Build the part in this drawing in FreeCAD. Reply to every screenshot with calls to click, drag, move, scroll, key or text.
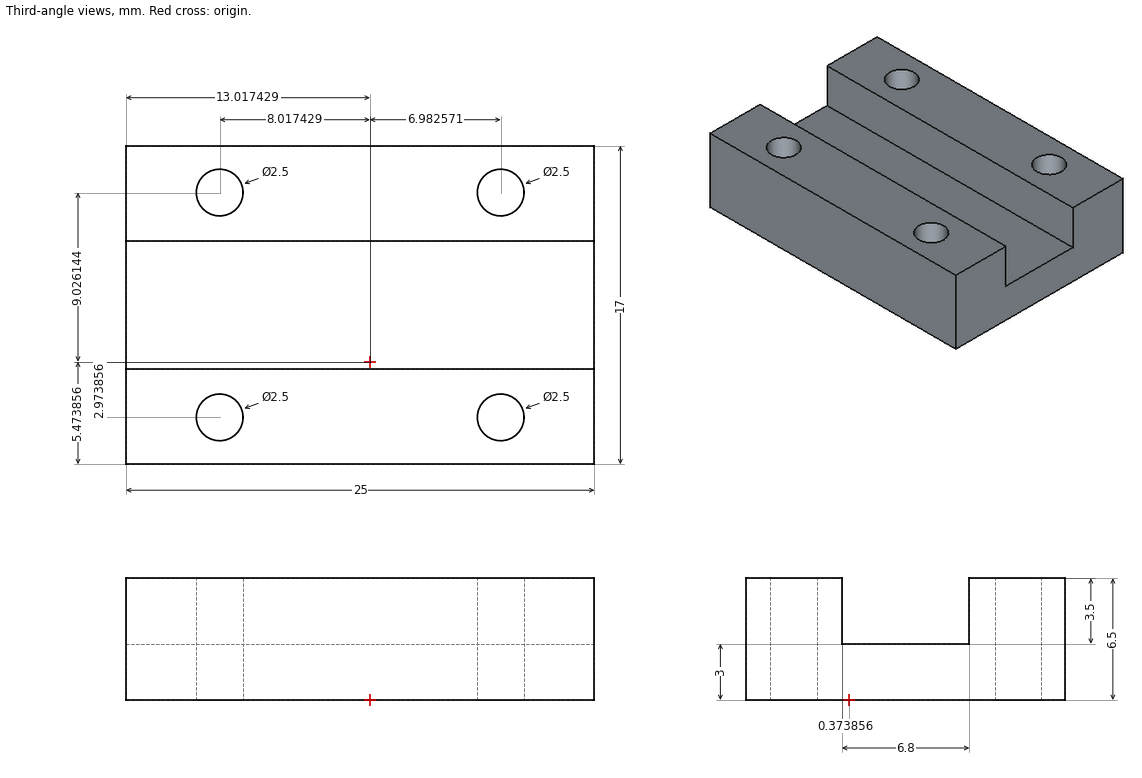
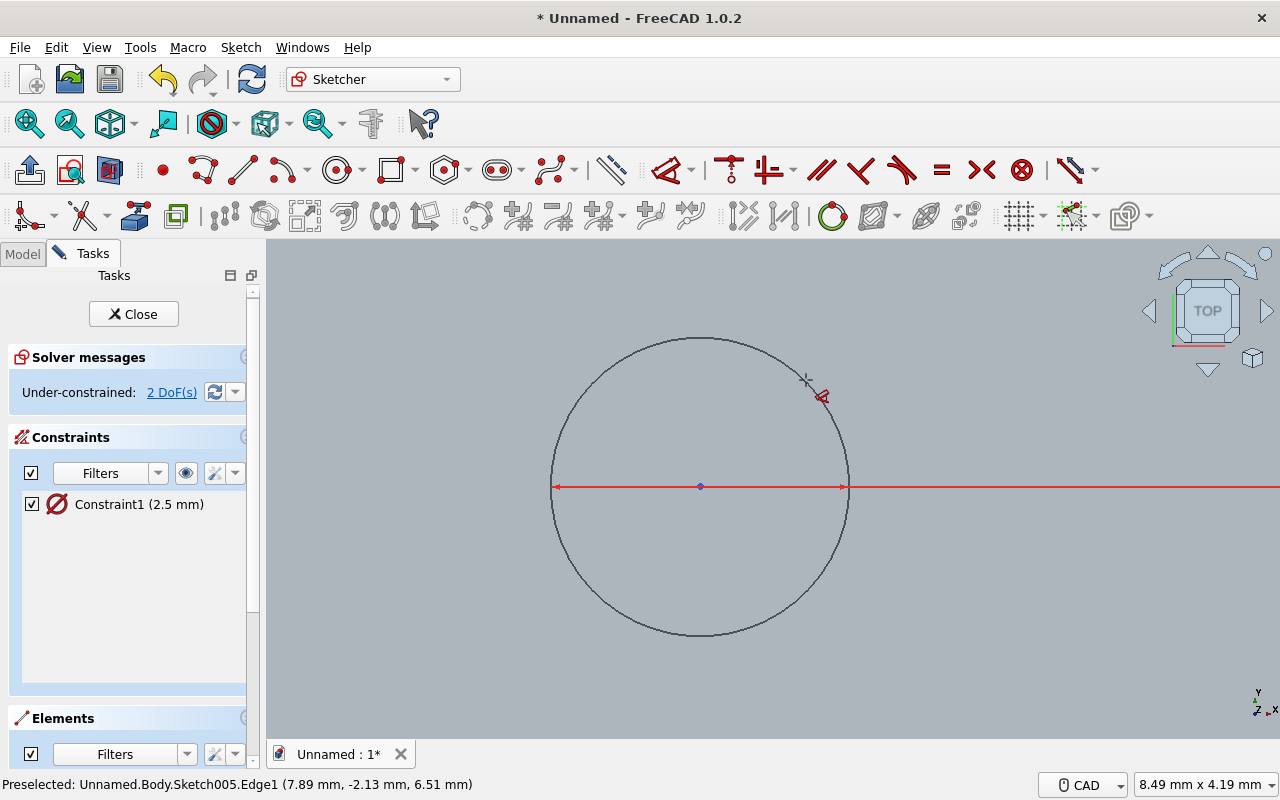
click(700, 487)
click(497, 521)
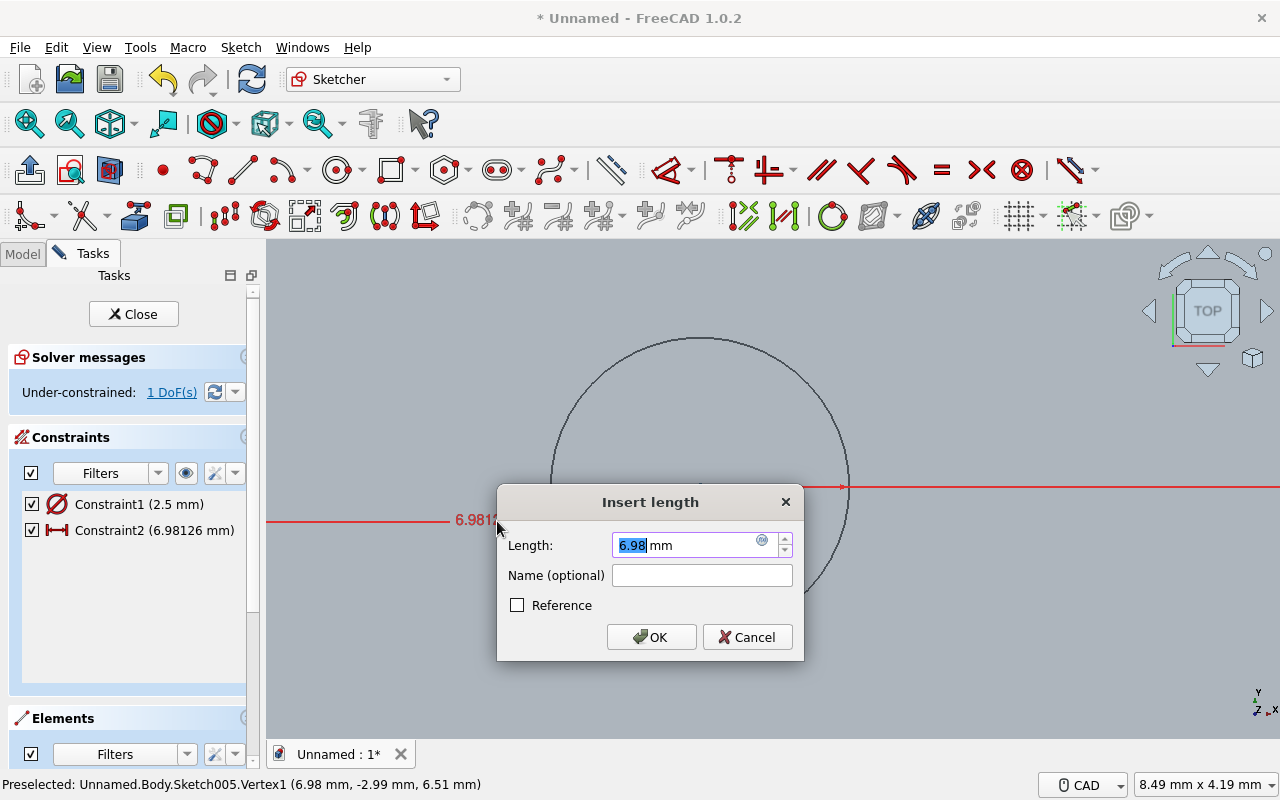
text(6.982571)
key(Return)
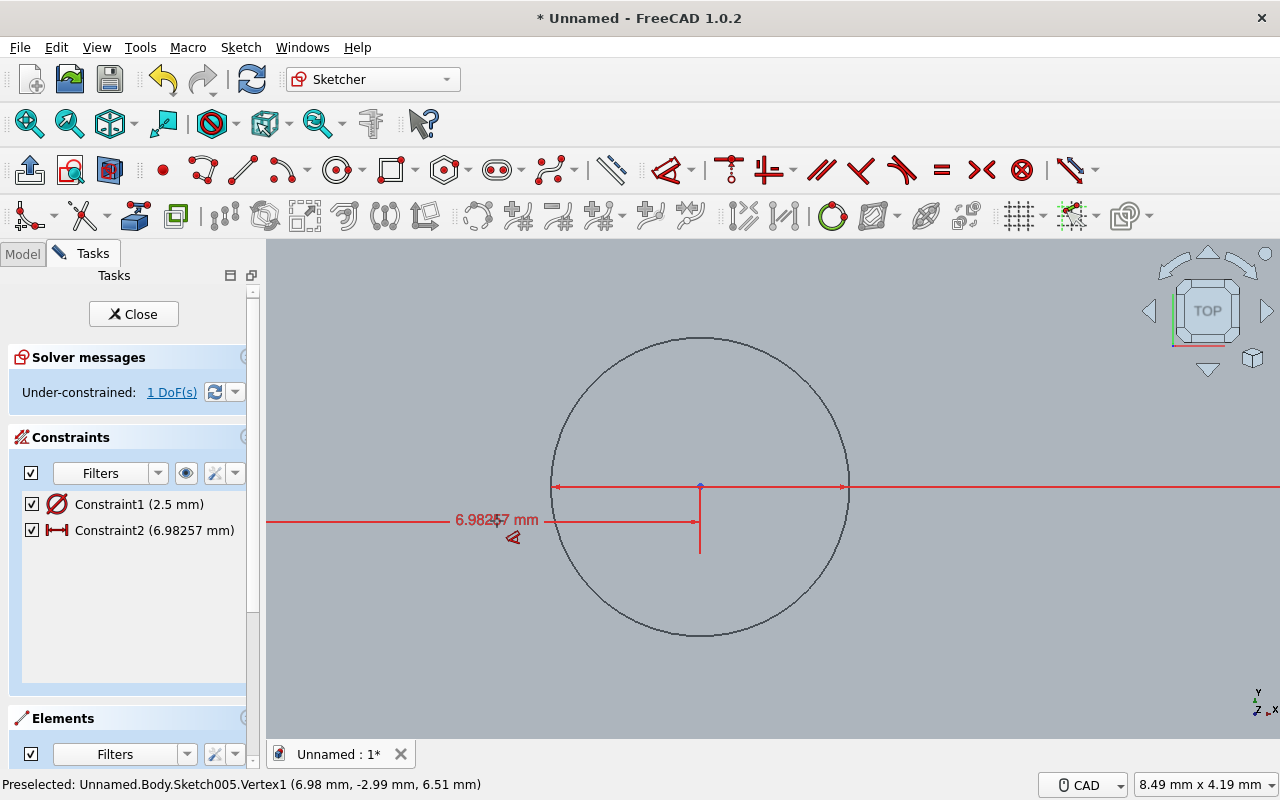
click(700, 487)
click(734, 377)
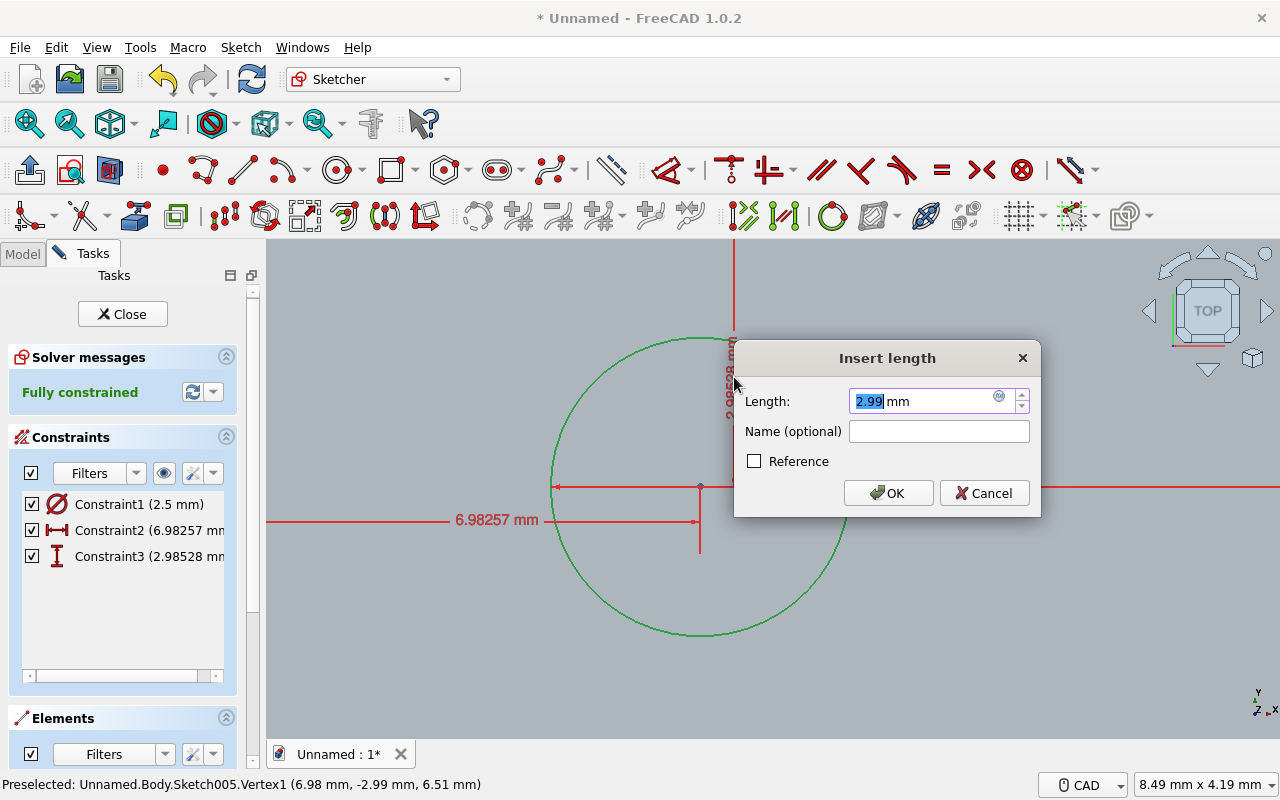
text(2.973856)
key(Return)
key(Escape)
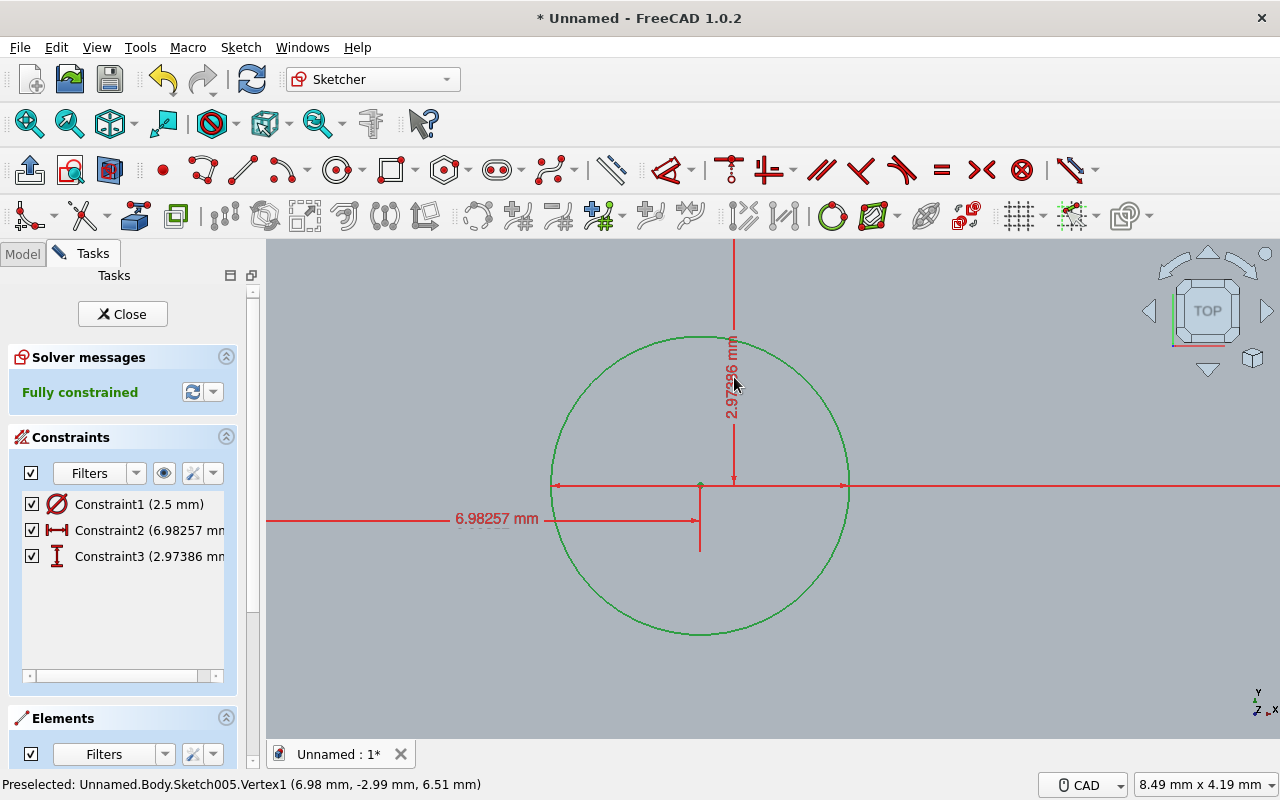
click(123, 314)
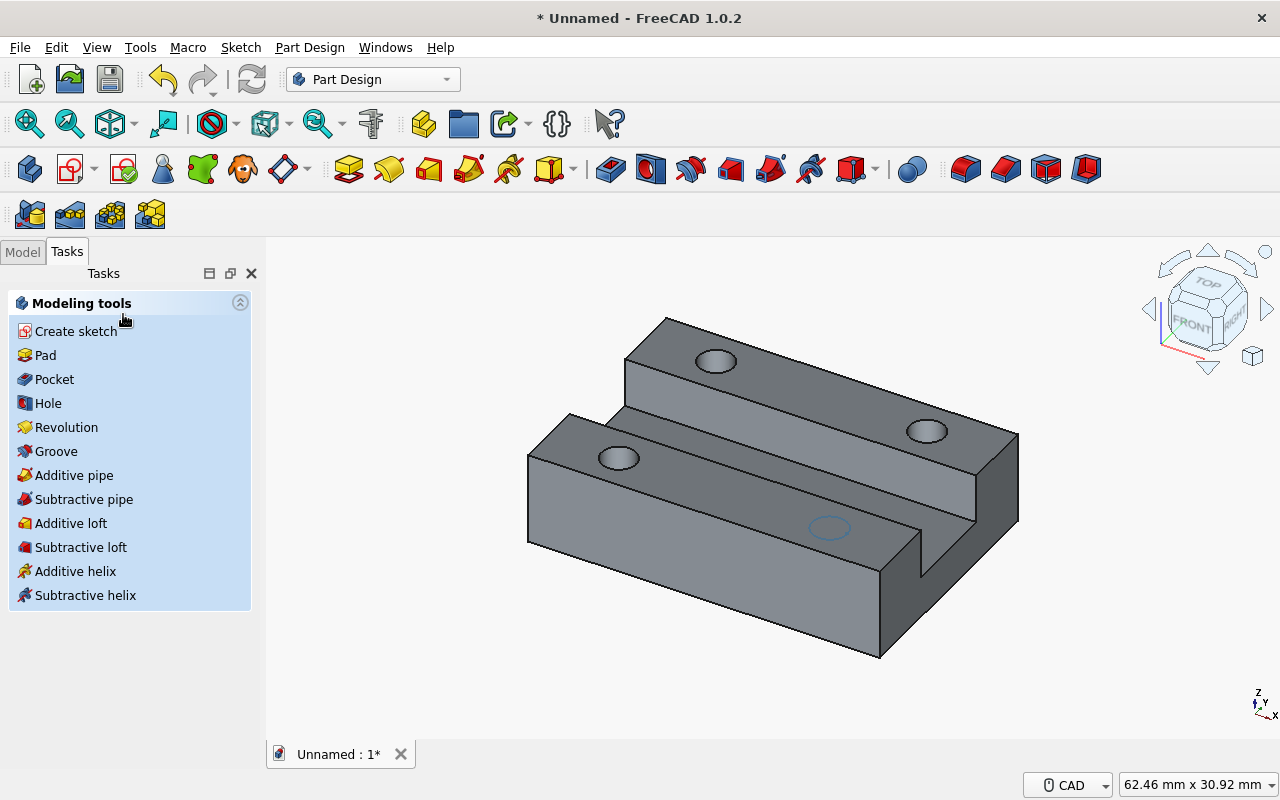
click(612, 170)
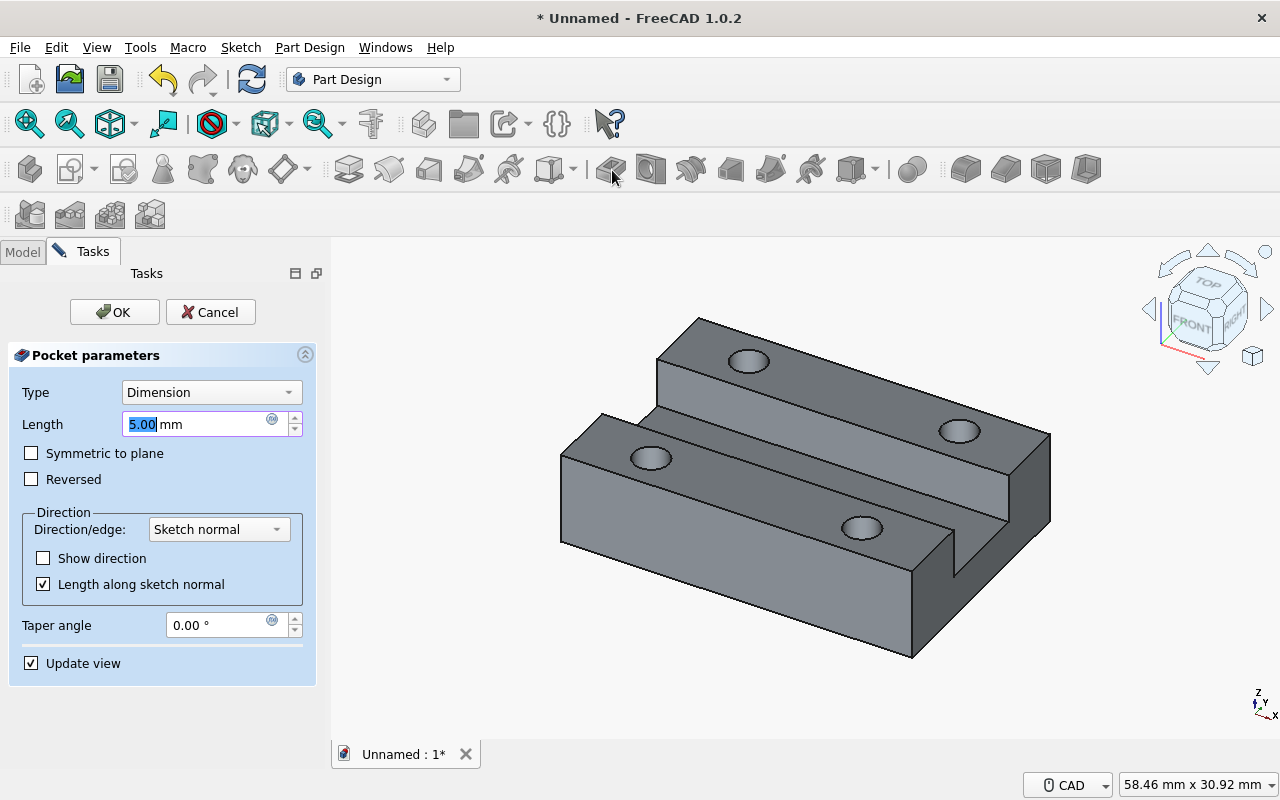
click(212, 392)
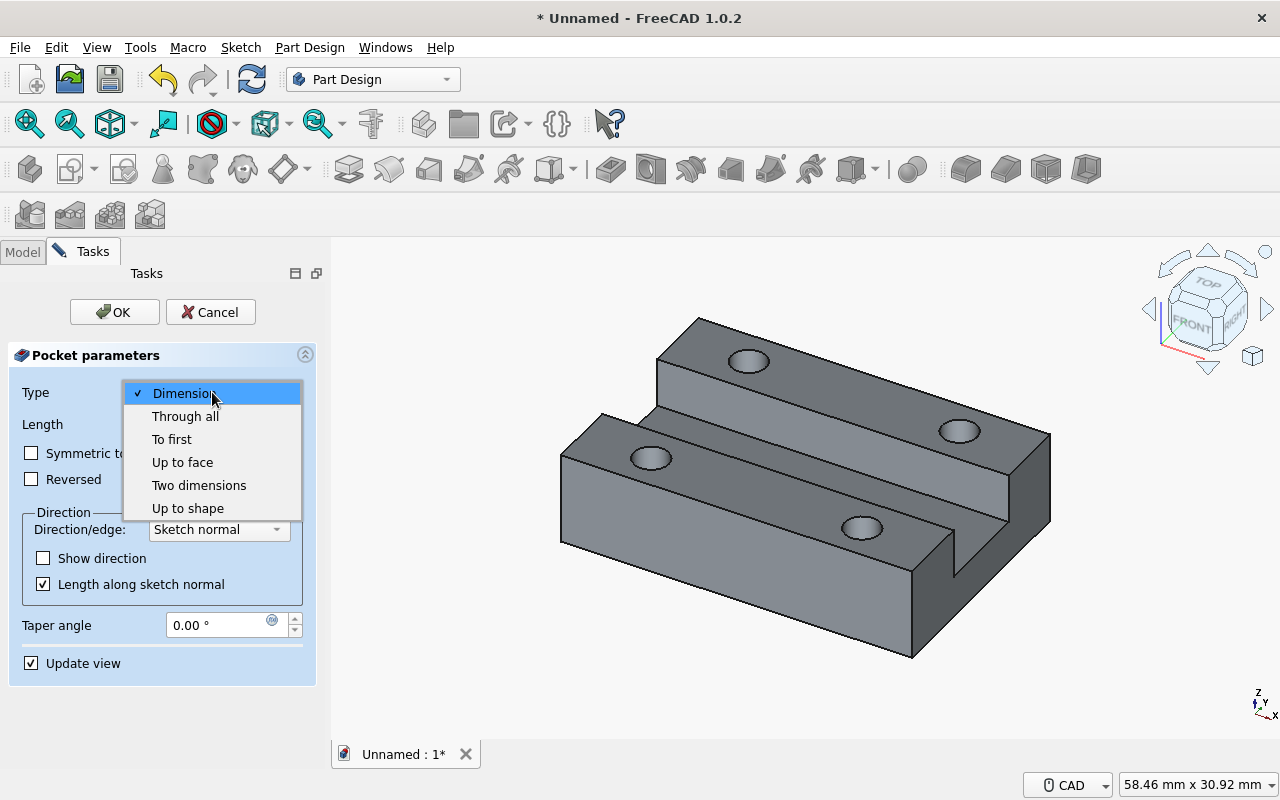
click(212, 440)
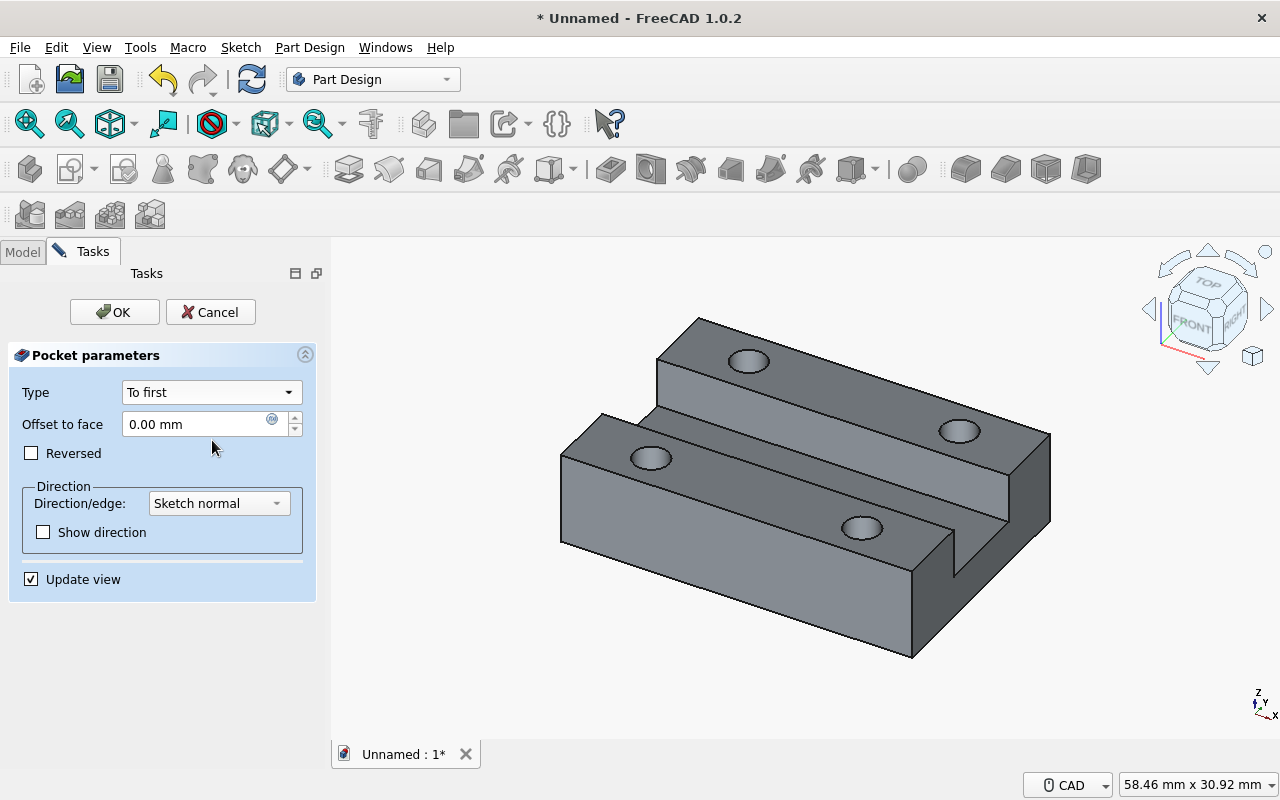
click(115, 312)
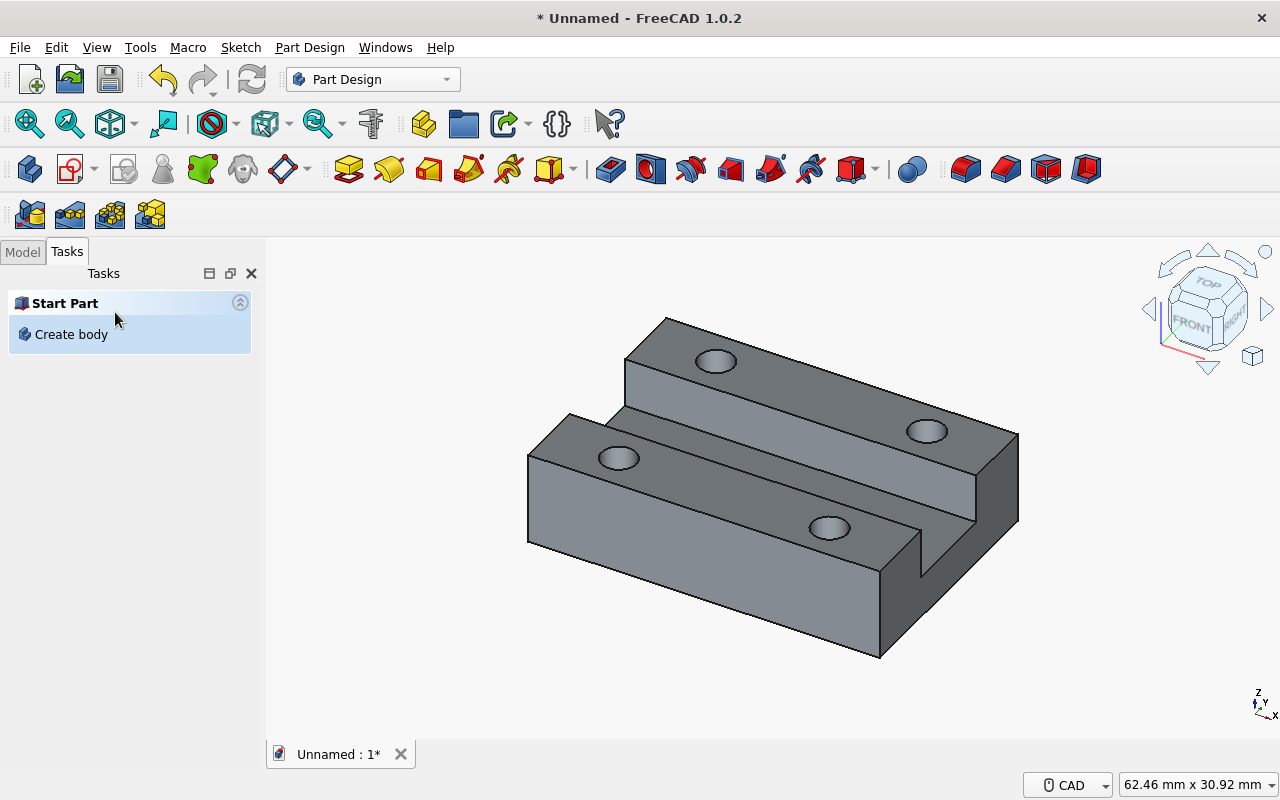
key(0)